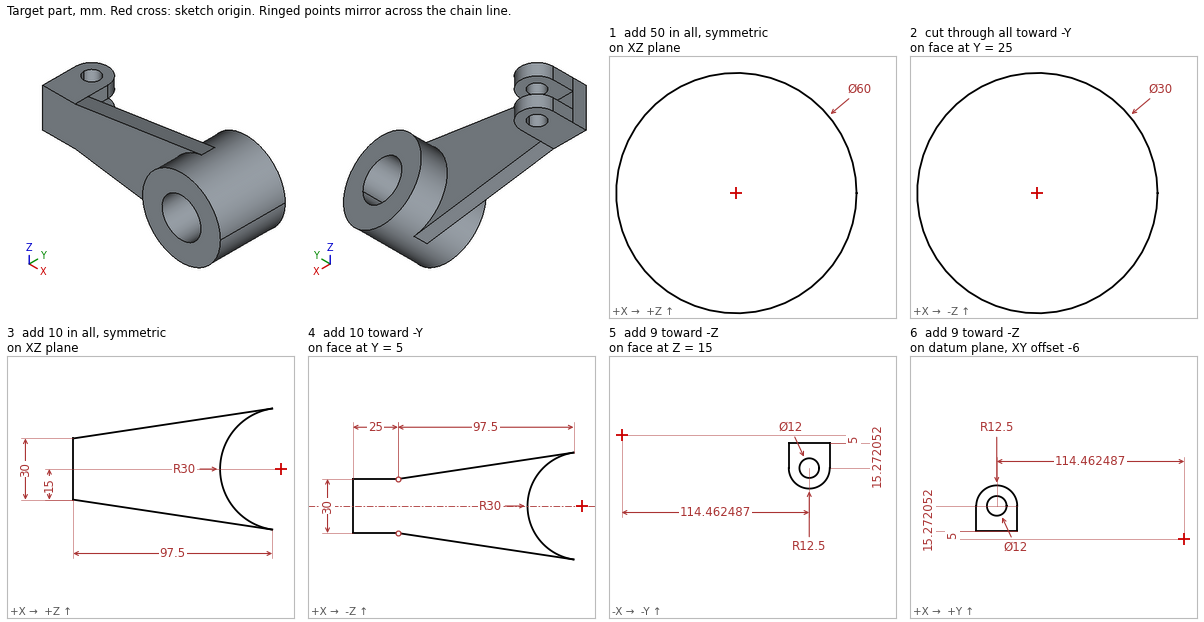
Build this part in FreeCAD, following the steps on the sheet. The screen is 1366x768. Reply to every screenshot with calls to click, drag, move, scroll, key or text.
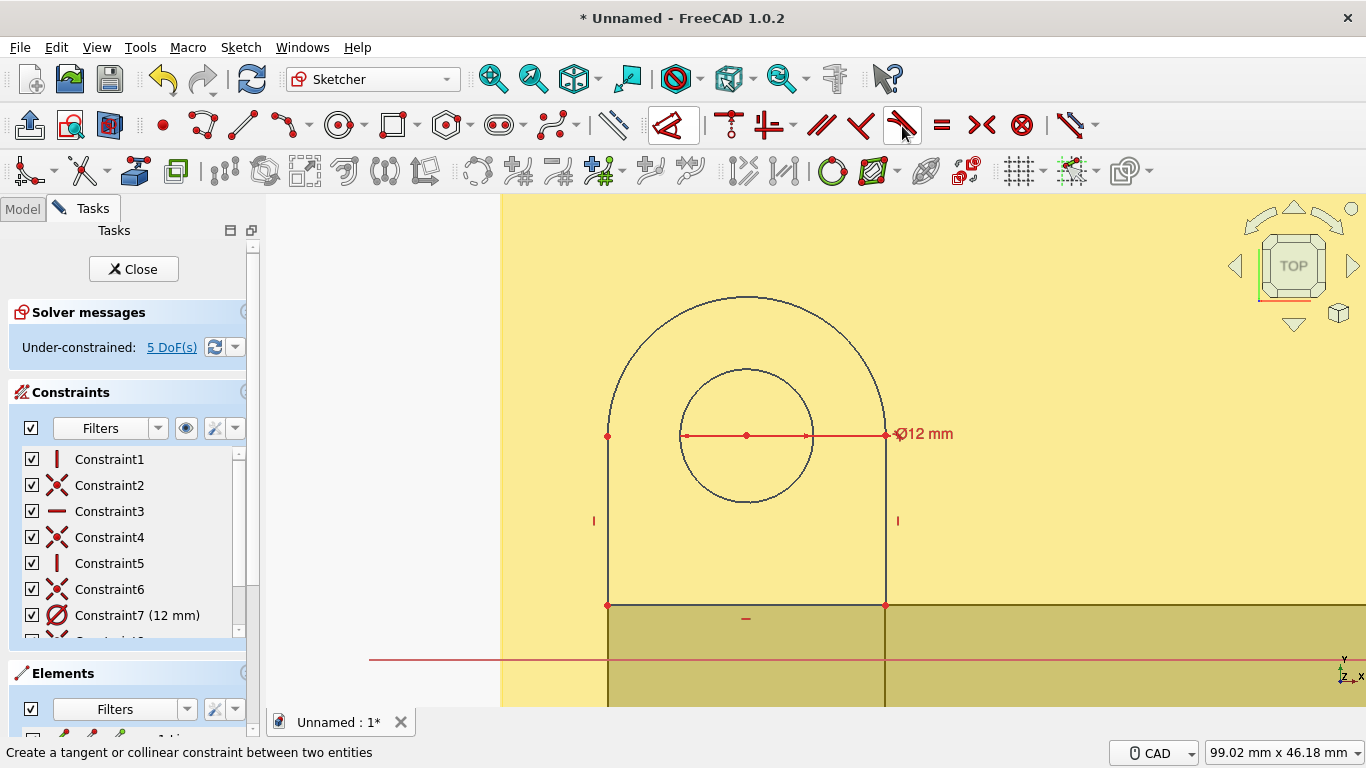
click(608, 555)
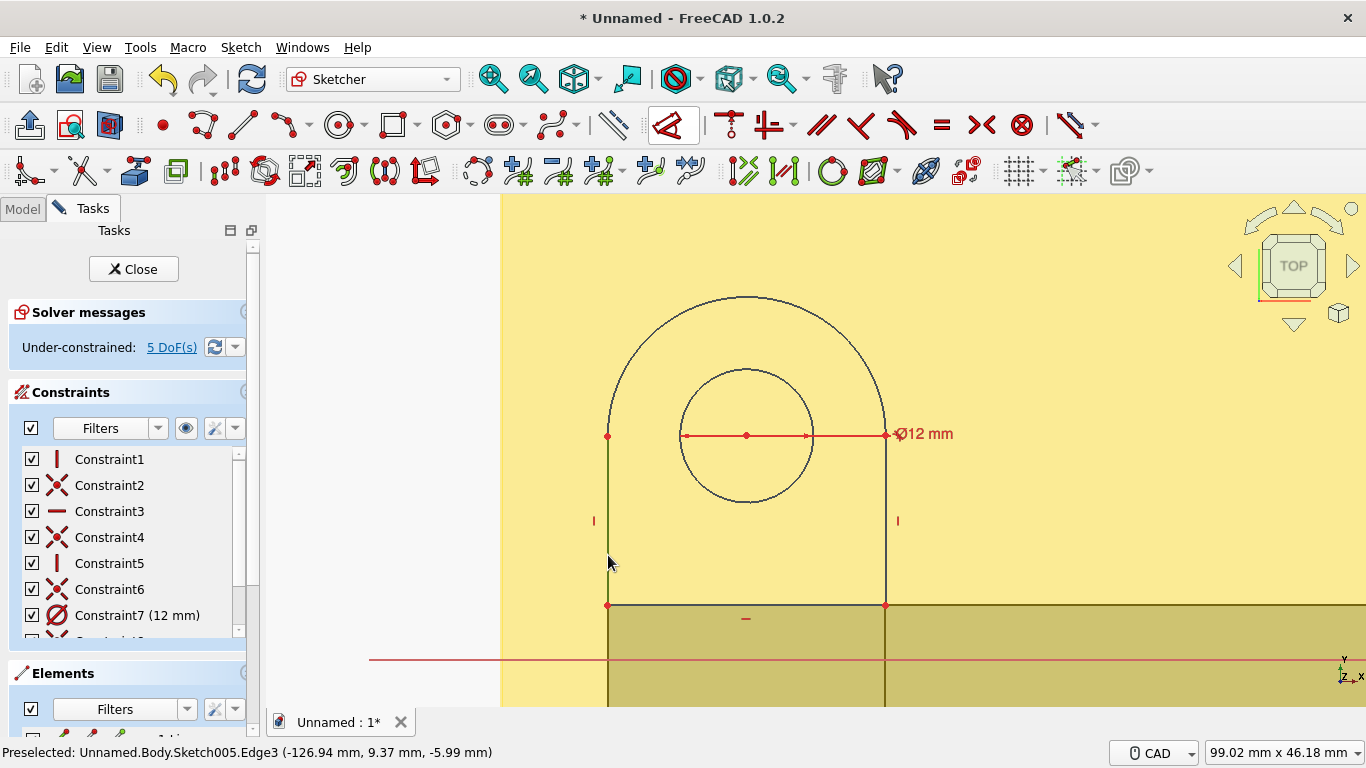
click(828, 324)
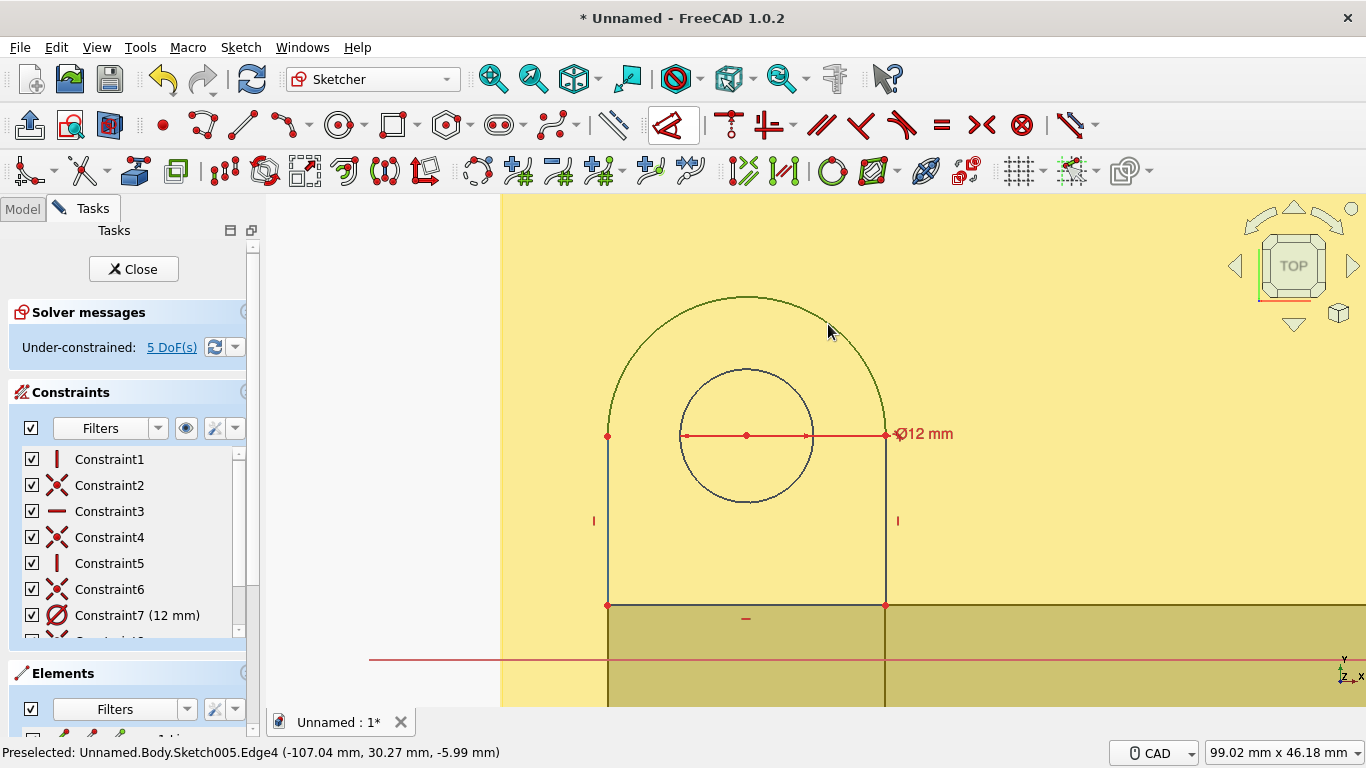
click(902, 126)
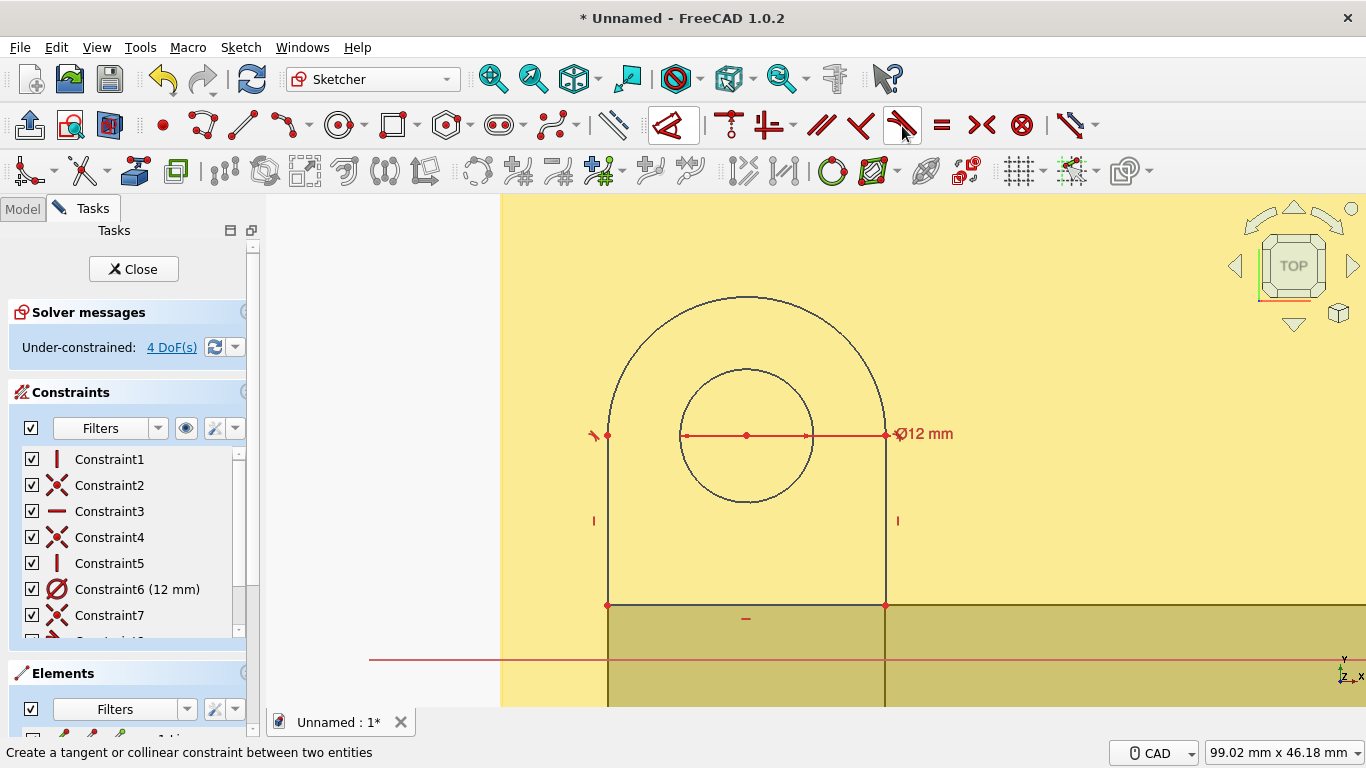
click(828, 324)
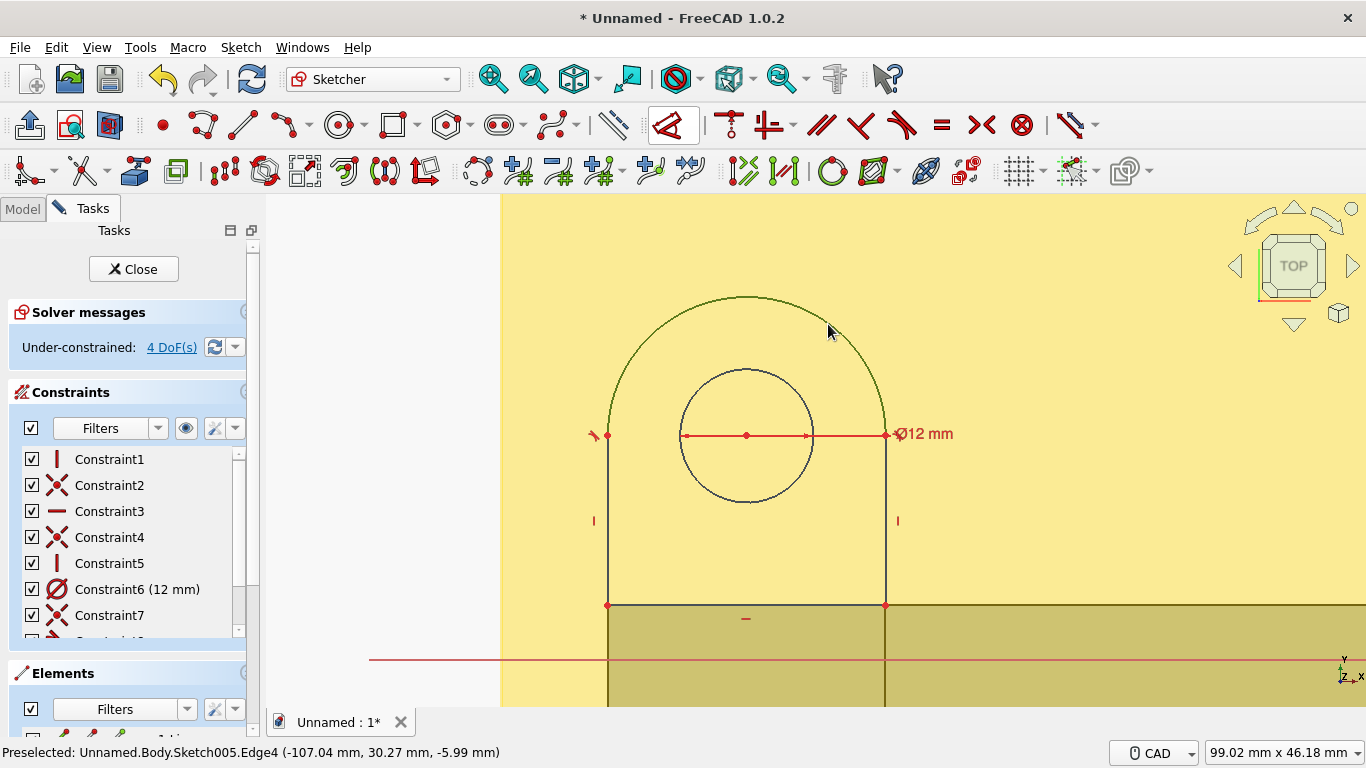
key(k)
key(r)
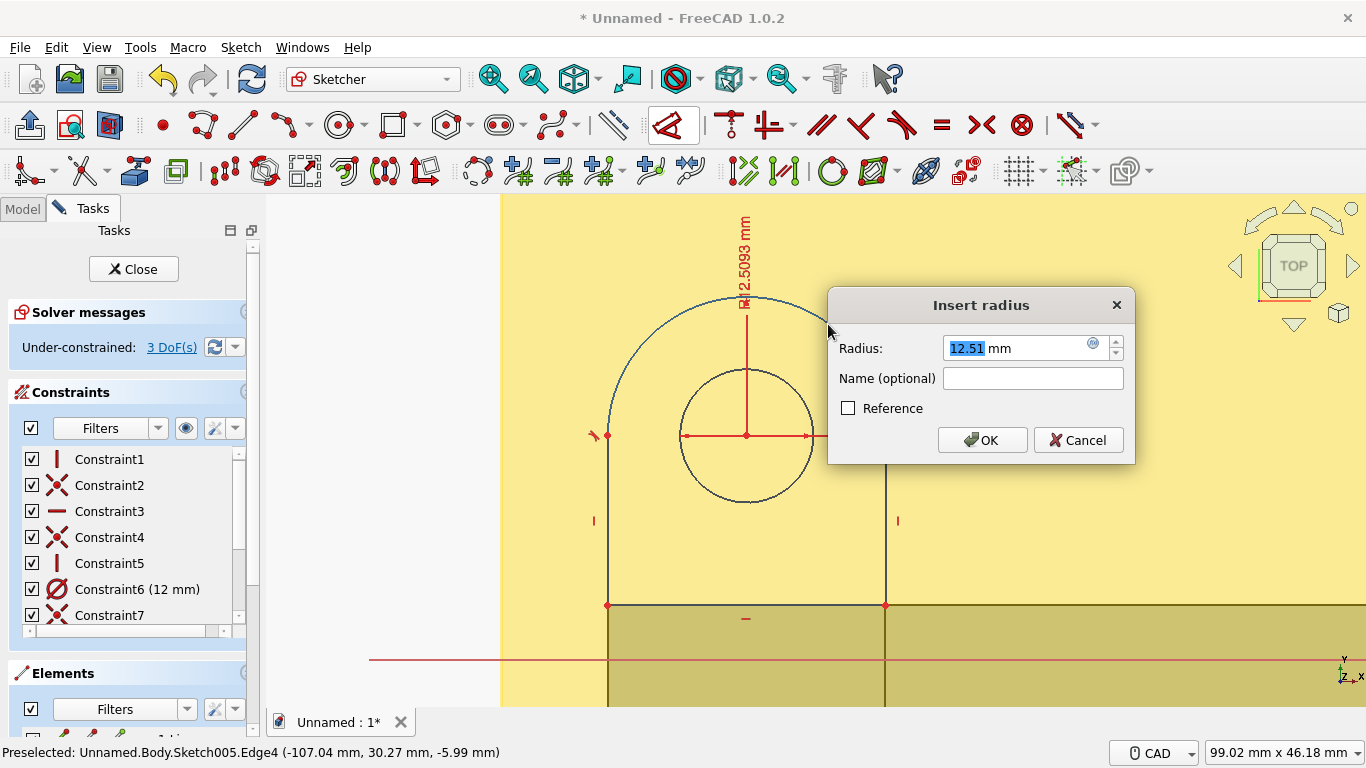
text(12.5)
key(Return)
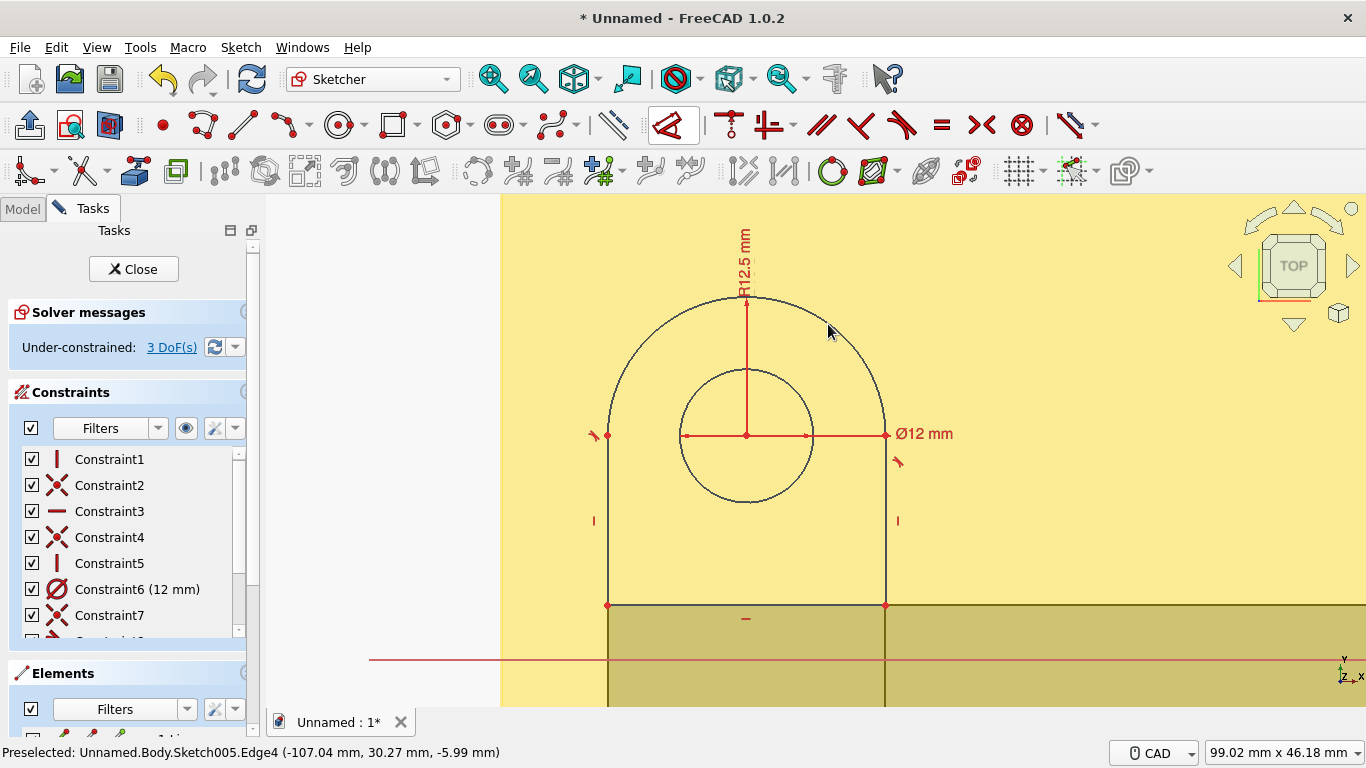
click(886, 605)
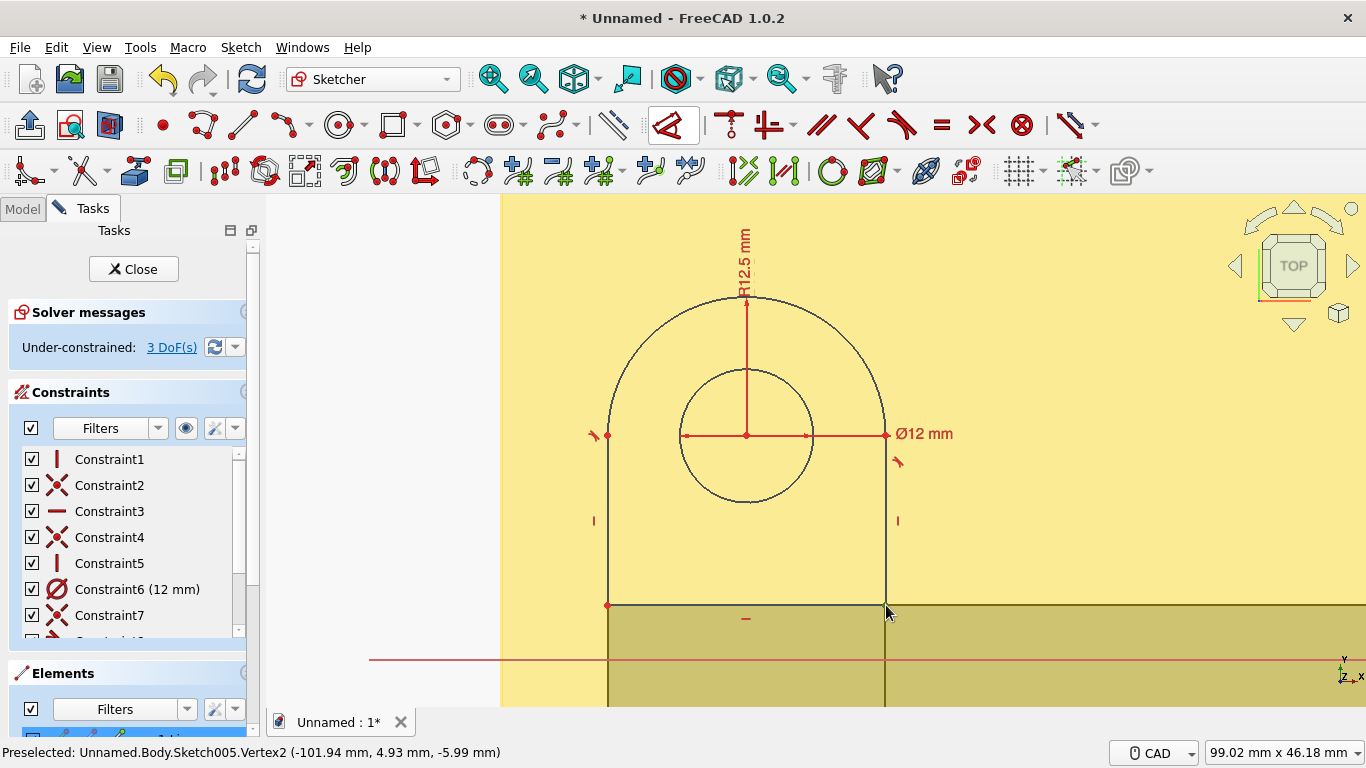
key(i)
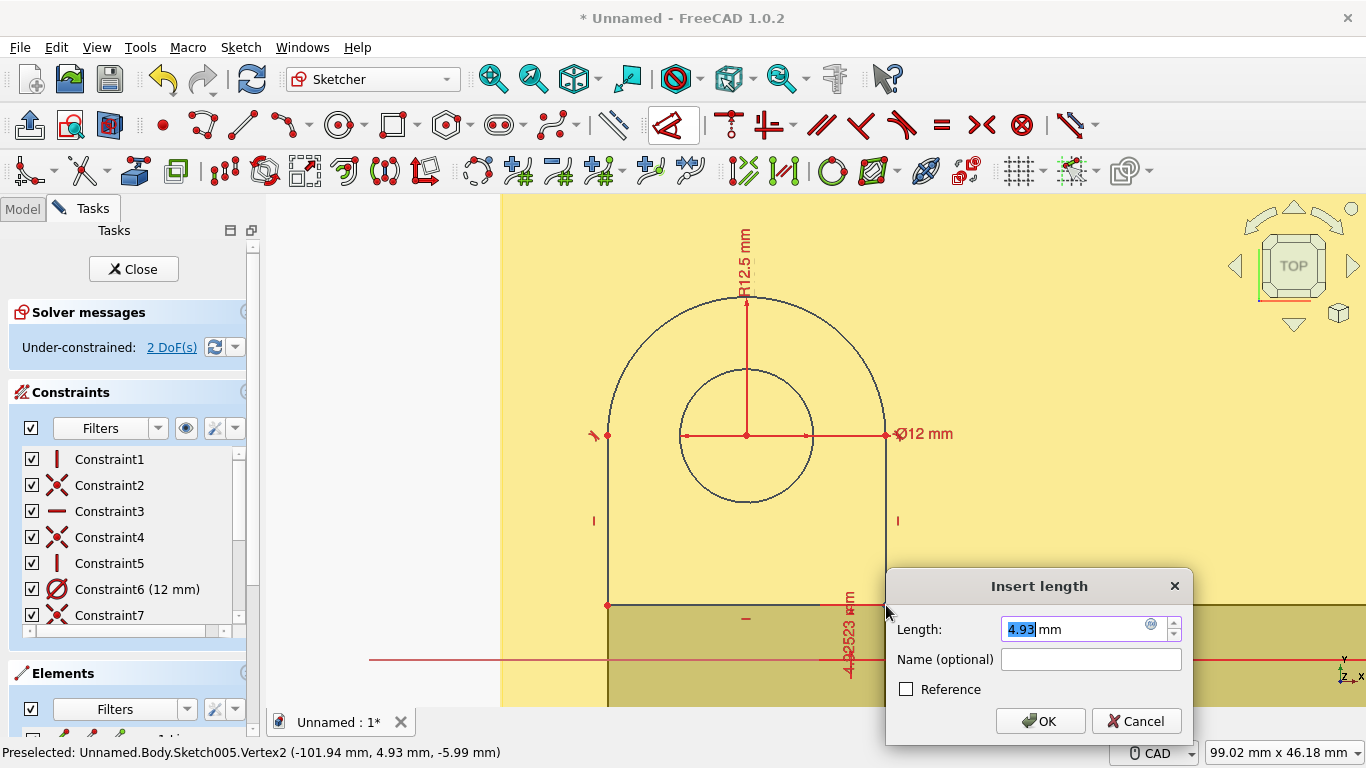
text(5)
key(Return)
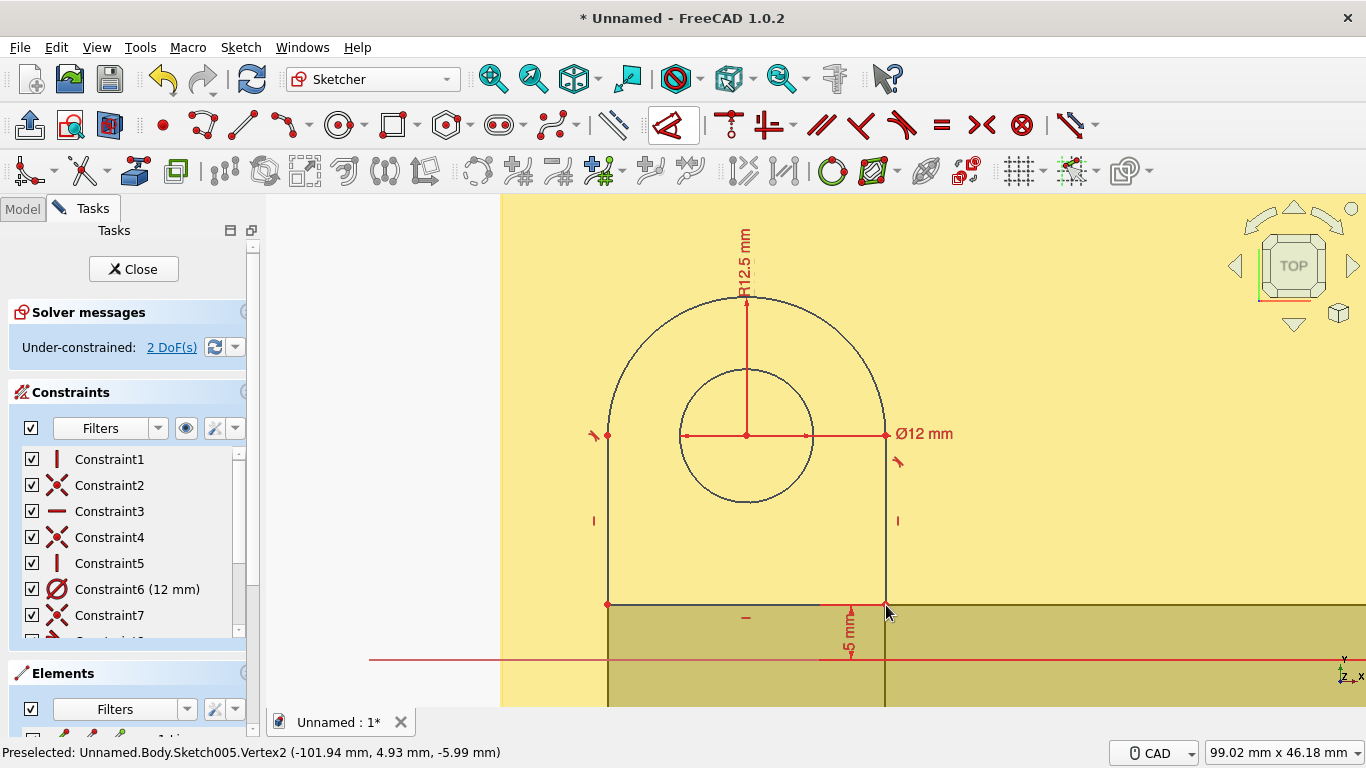
click(886, 487)